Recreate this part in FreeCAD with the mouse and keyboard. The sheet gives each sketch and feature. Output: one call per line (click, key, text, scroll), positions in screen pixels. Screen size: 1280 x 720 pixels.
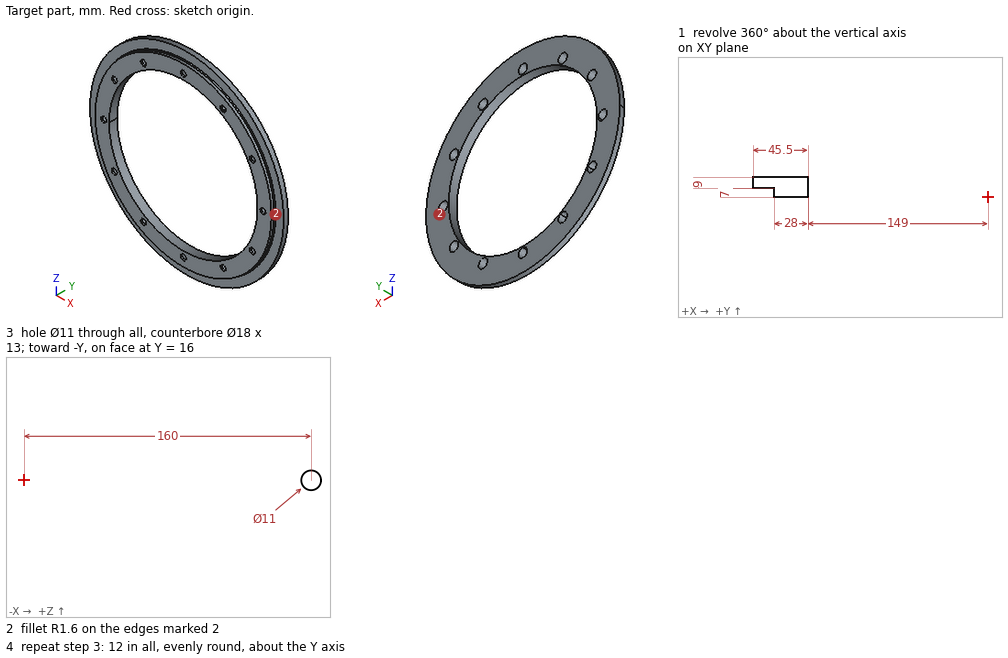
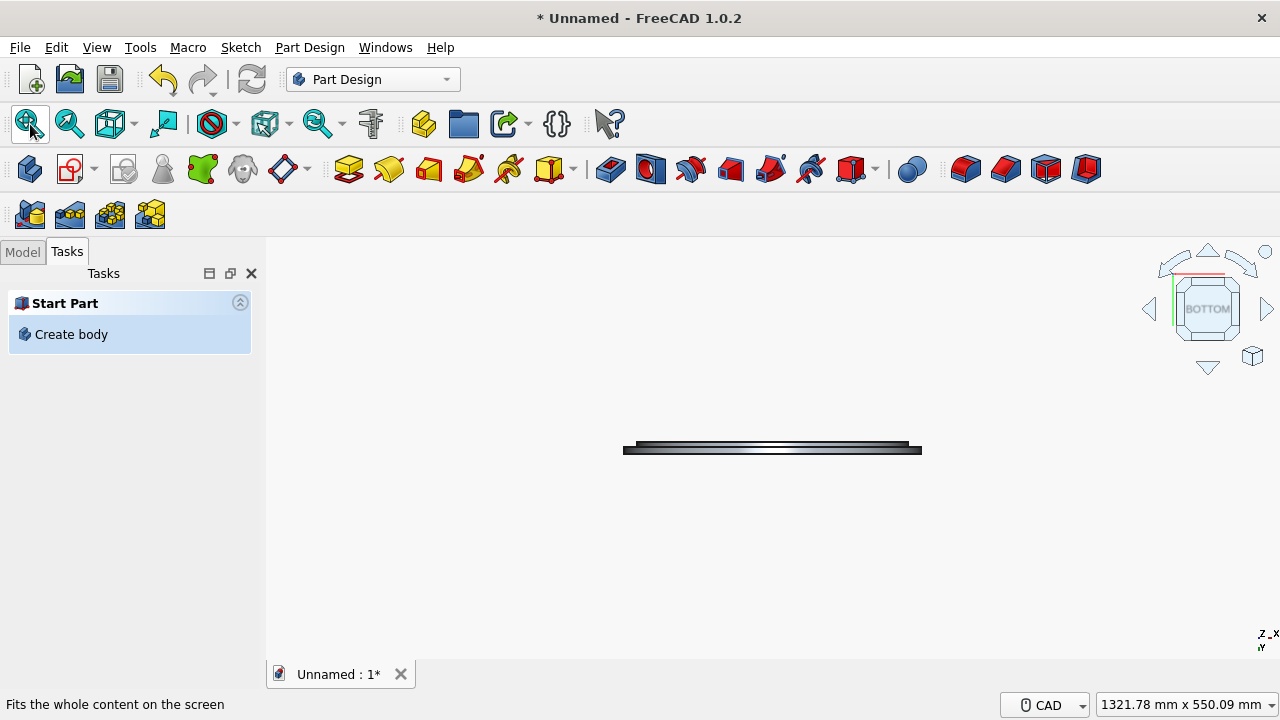
key(4)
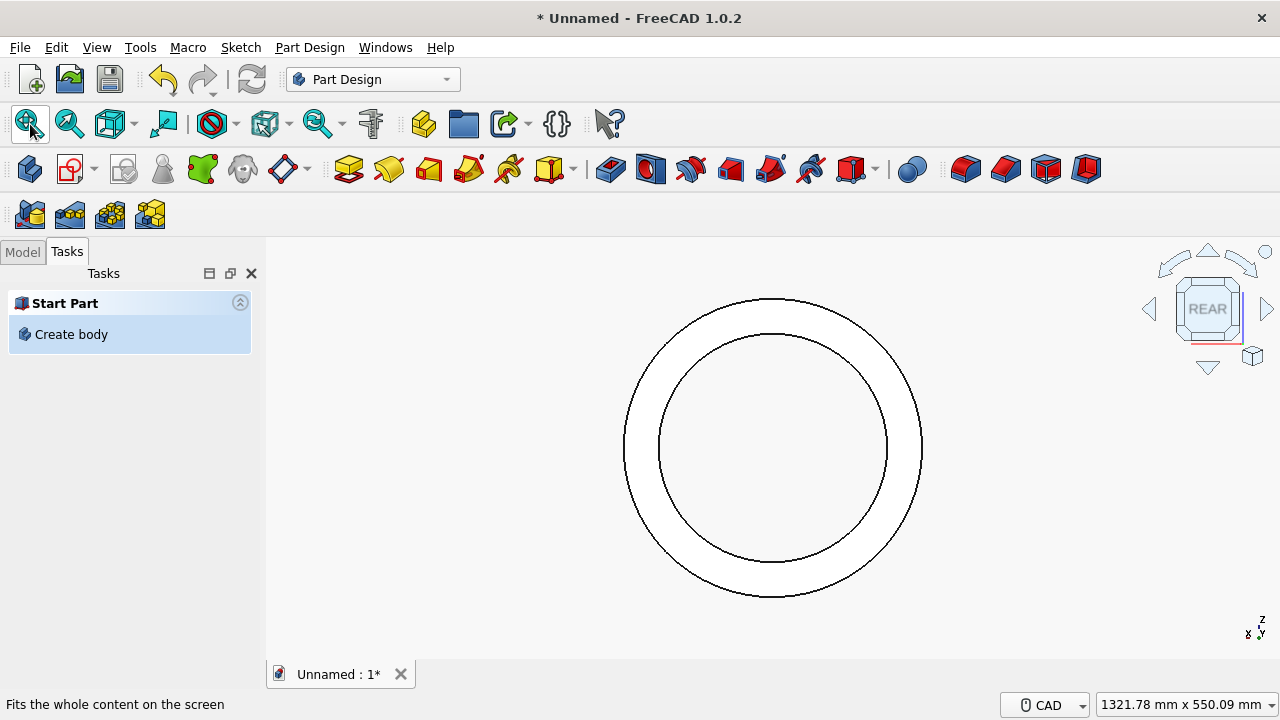
key(6)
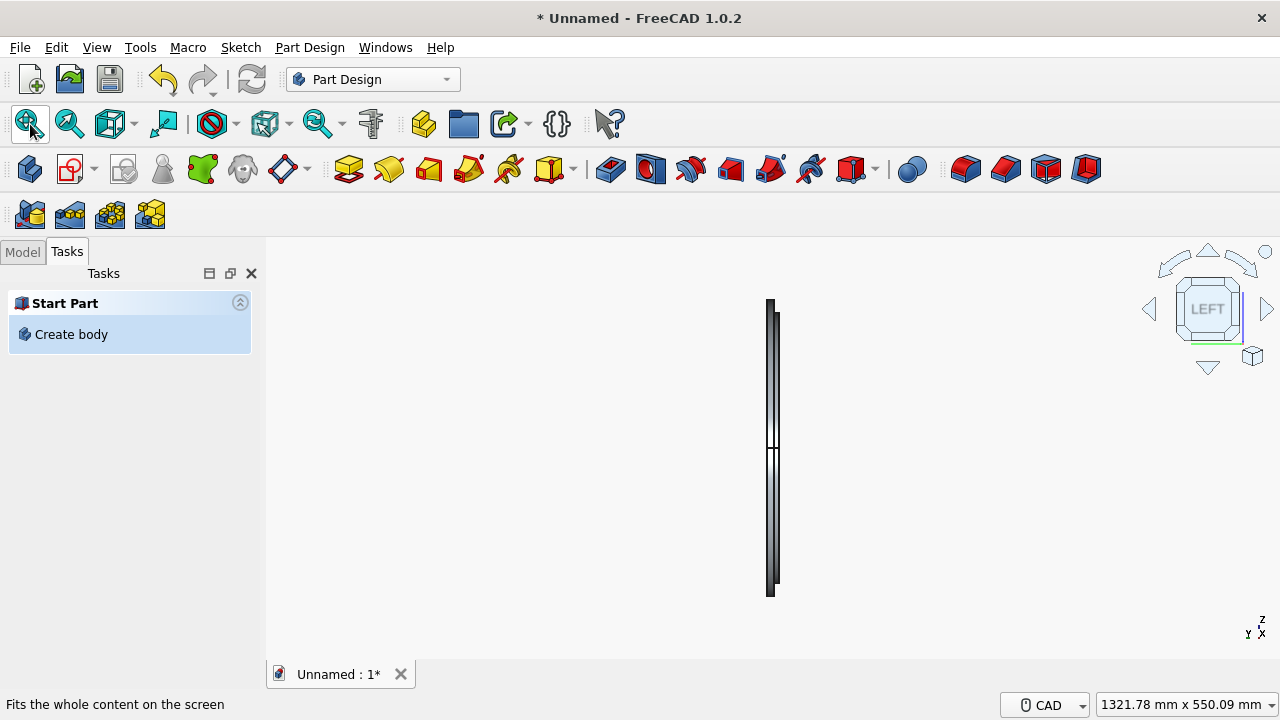
key(v)
key(3)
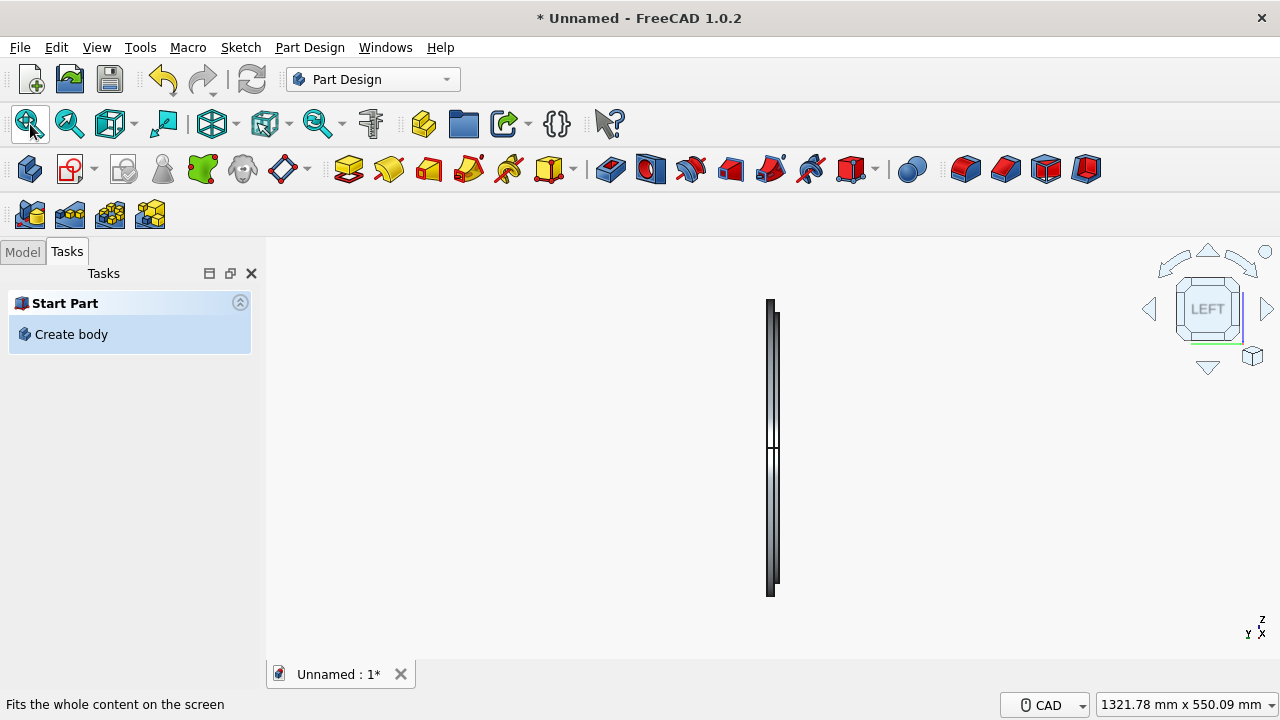
key(0)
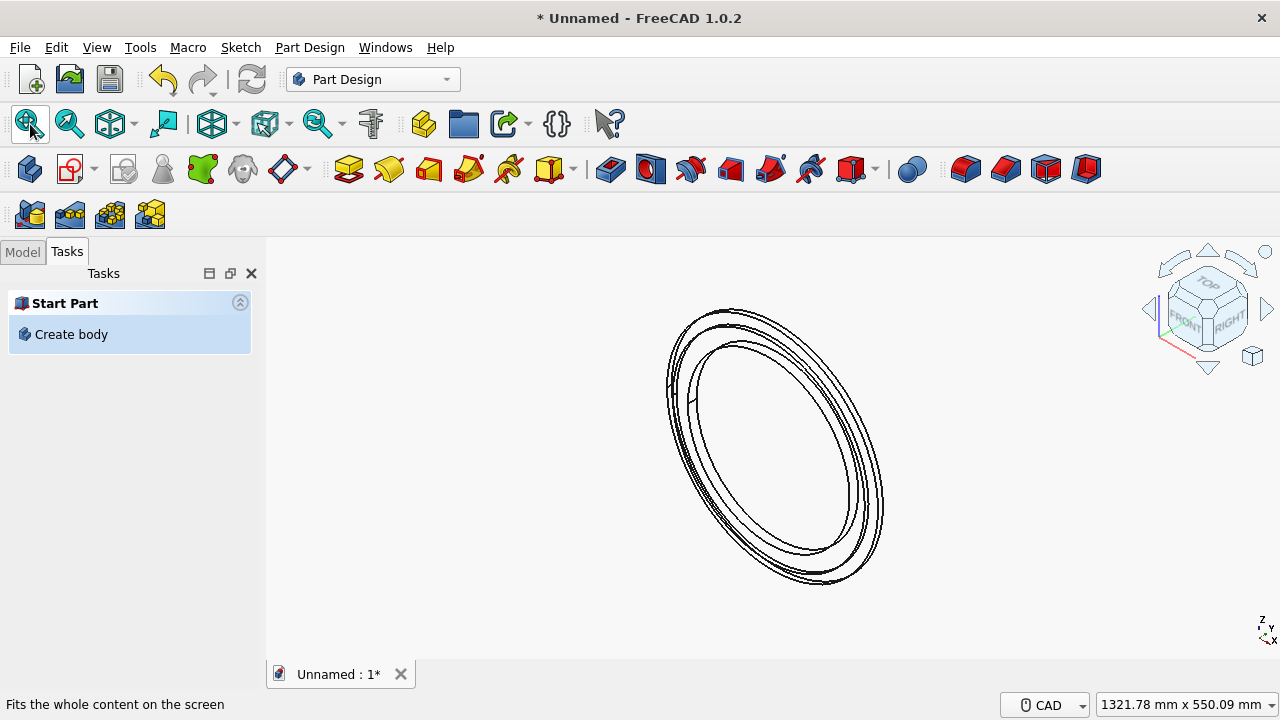
scroll(869, 503, up, 6)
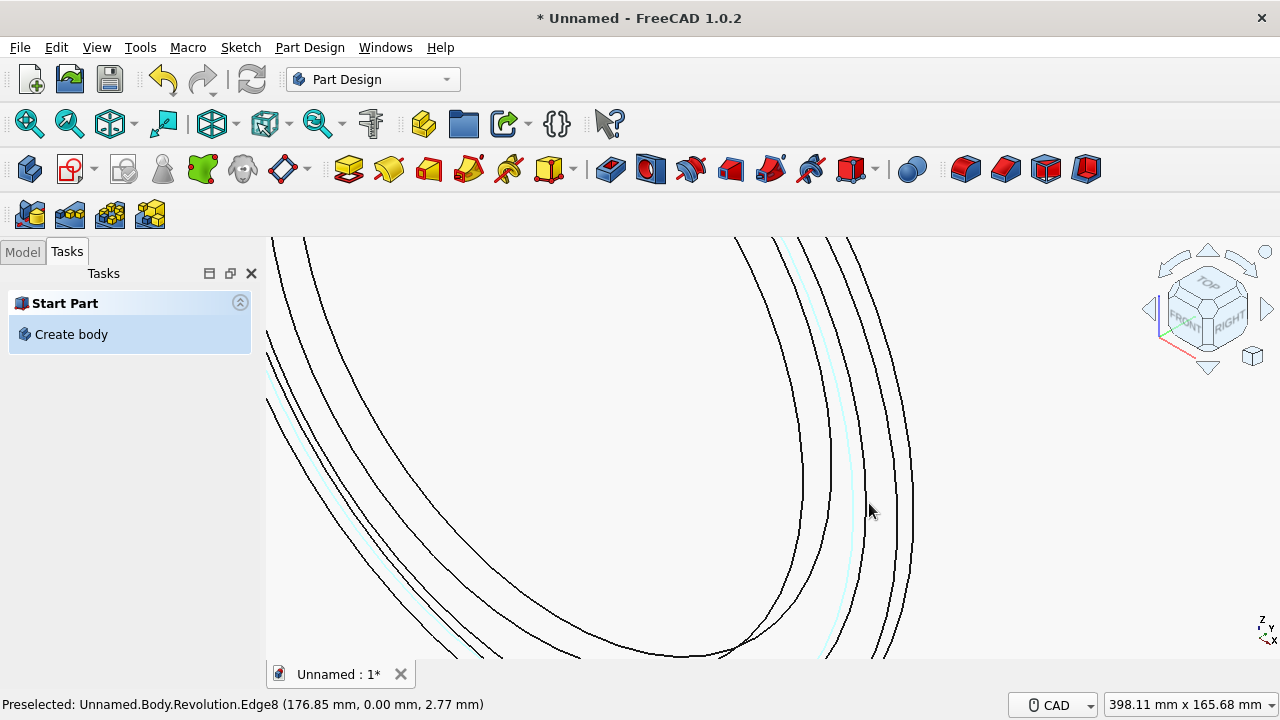
click(866, 503)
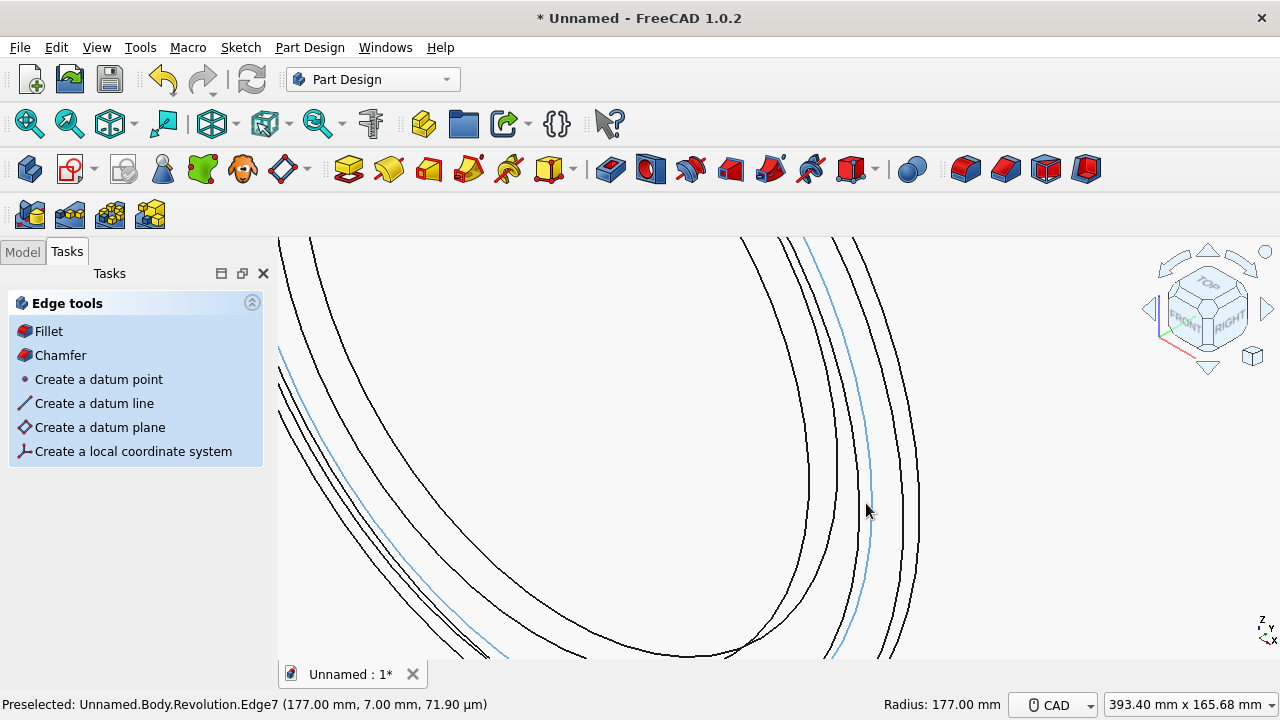
key(v)
key(1)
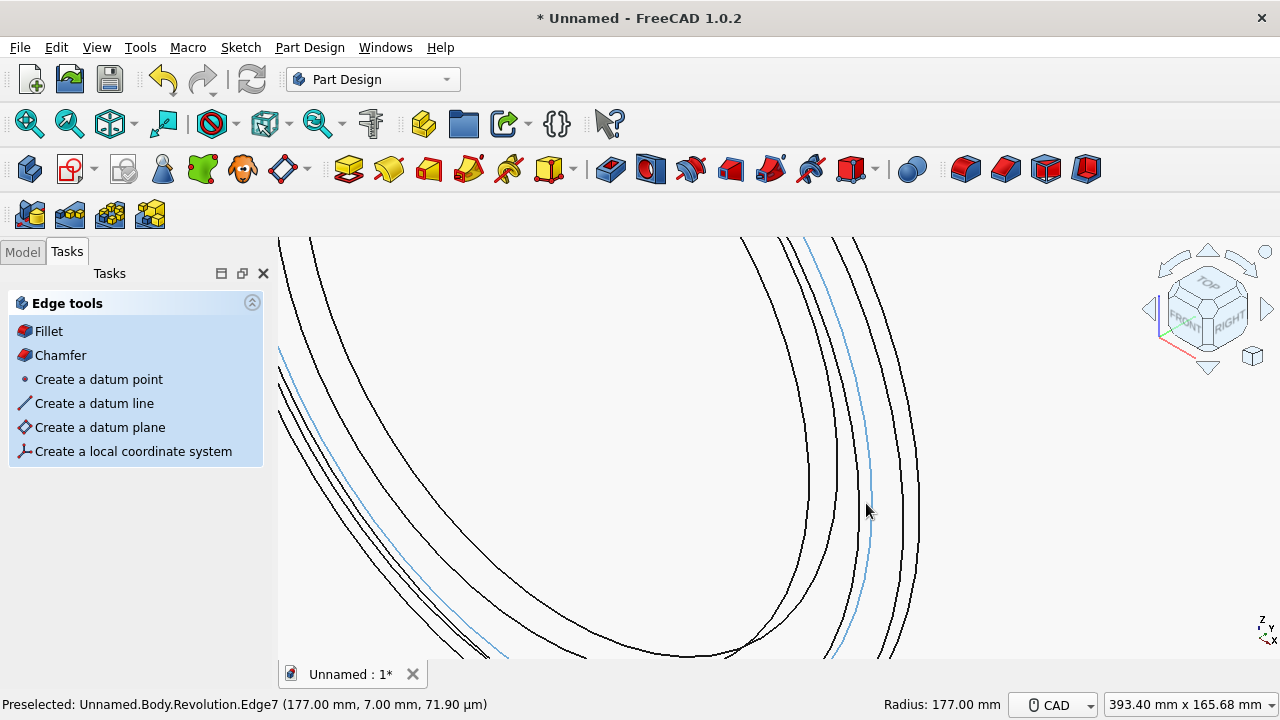
click(966, 170)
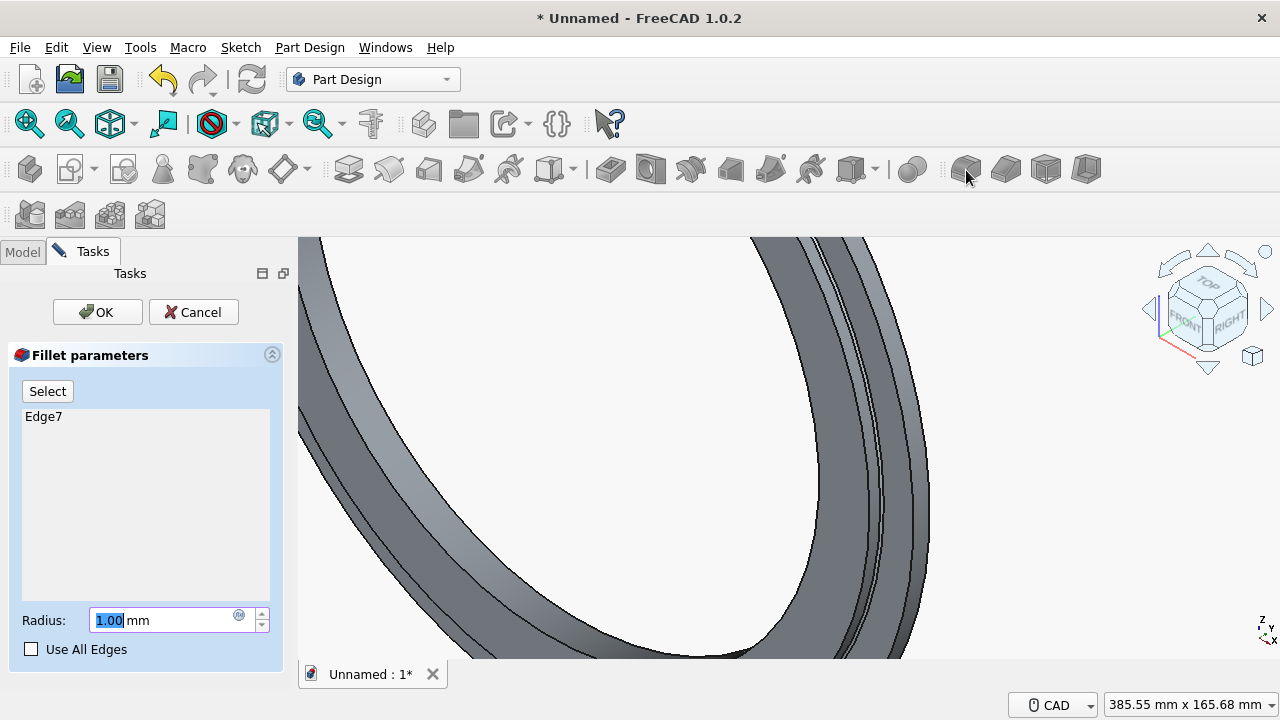
text(1.6)
key(Tab)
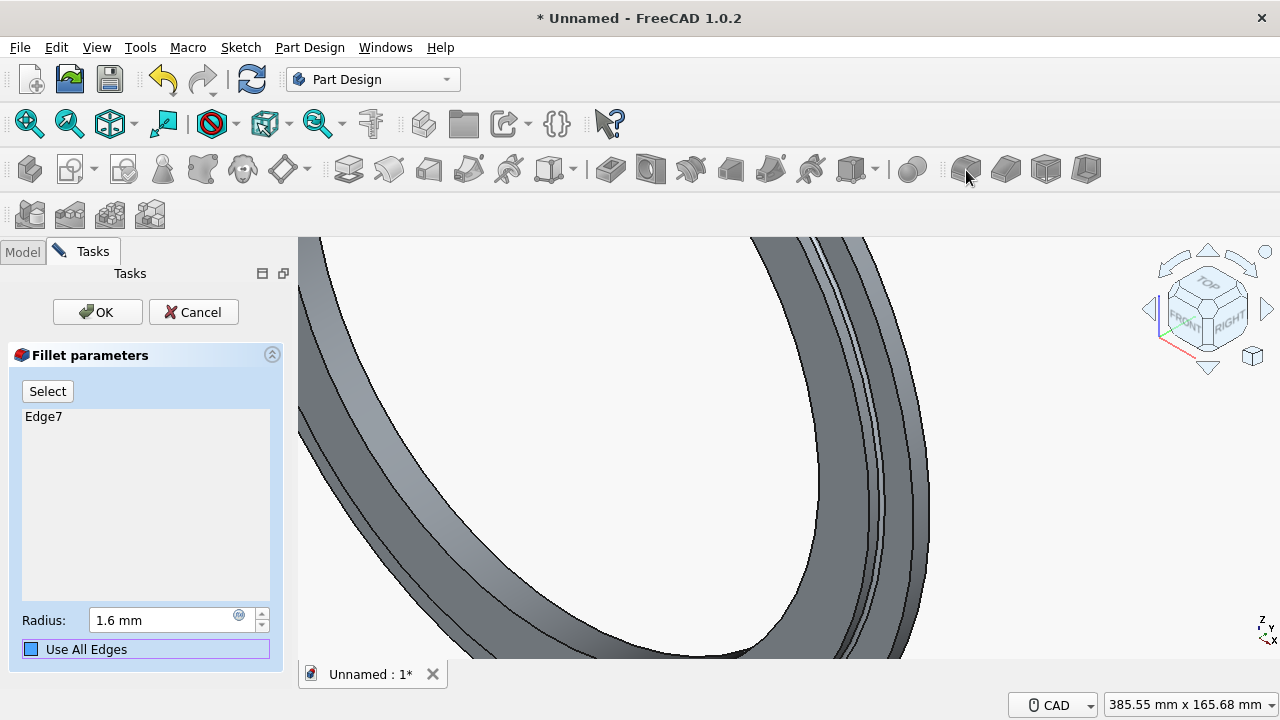
click(98, 312)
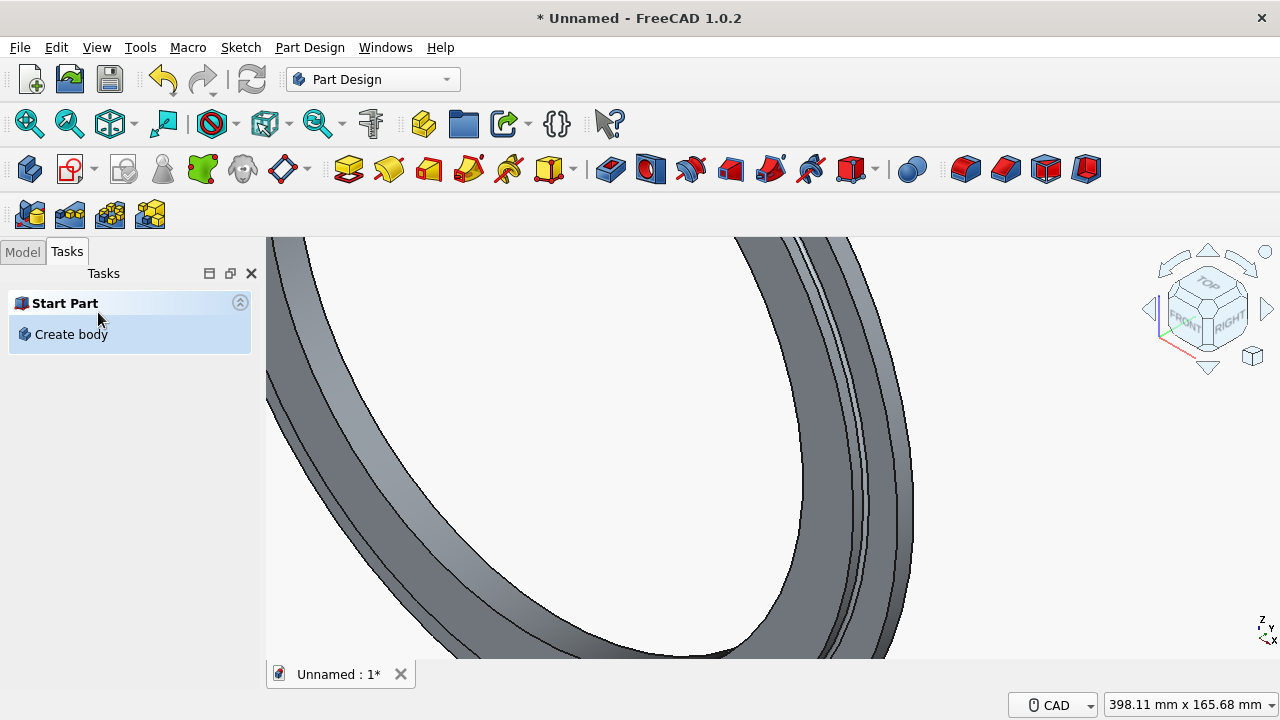
click(30, 124)